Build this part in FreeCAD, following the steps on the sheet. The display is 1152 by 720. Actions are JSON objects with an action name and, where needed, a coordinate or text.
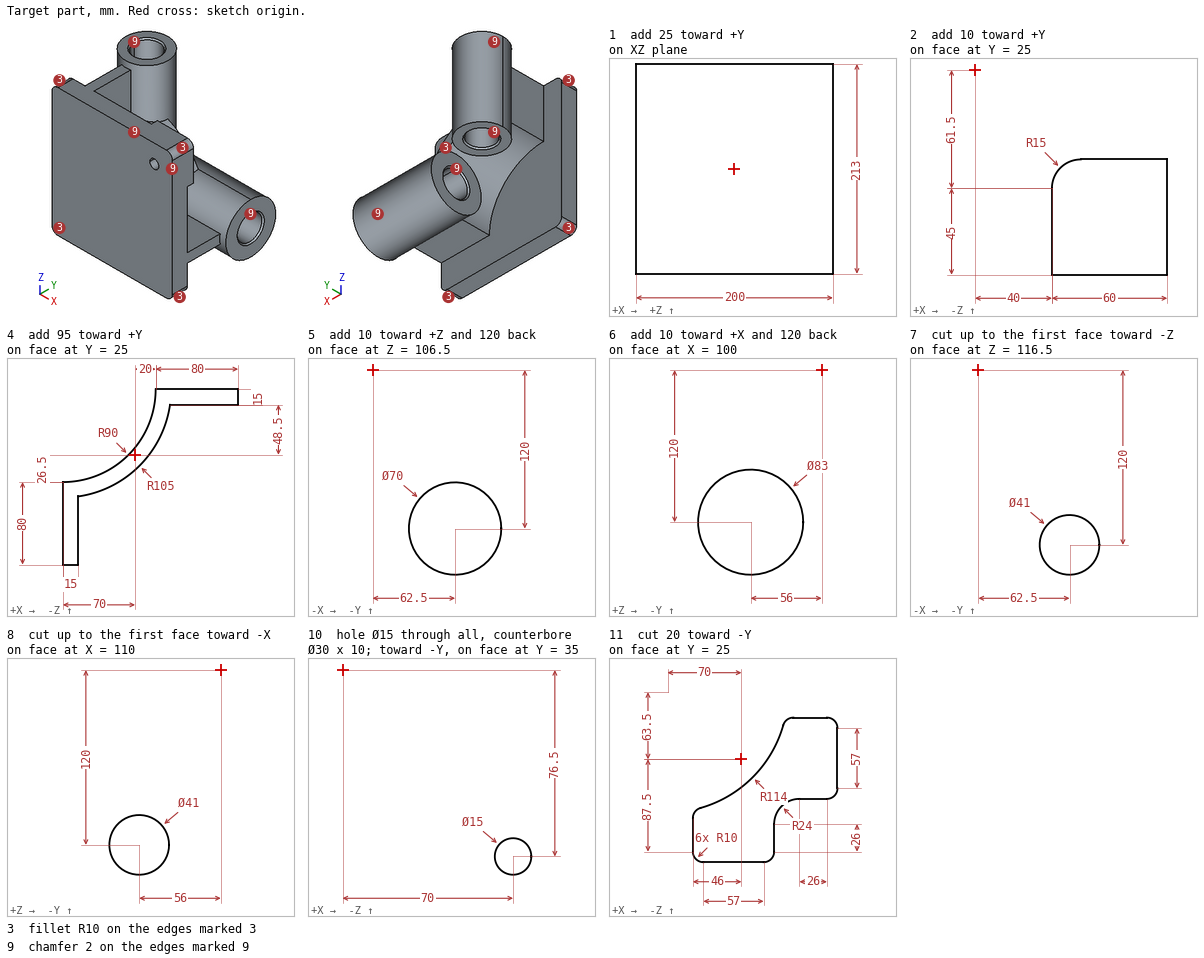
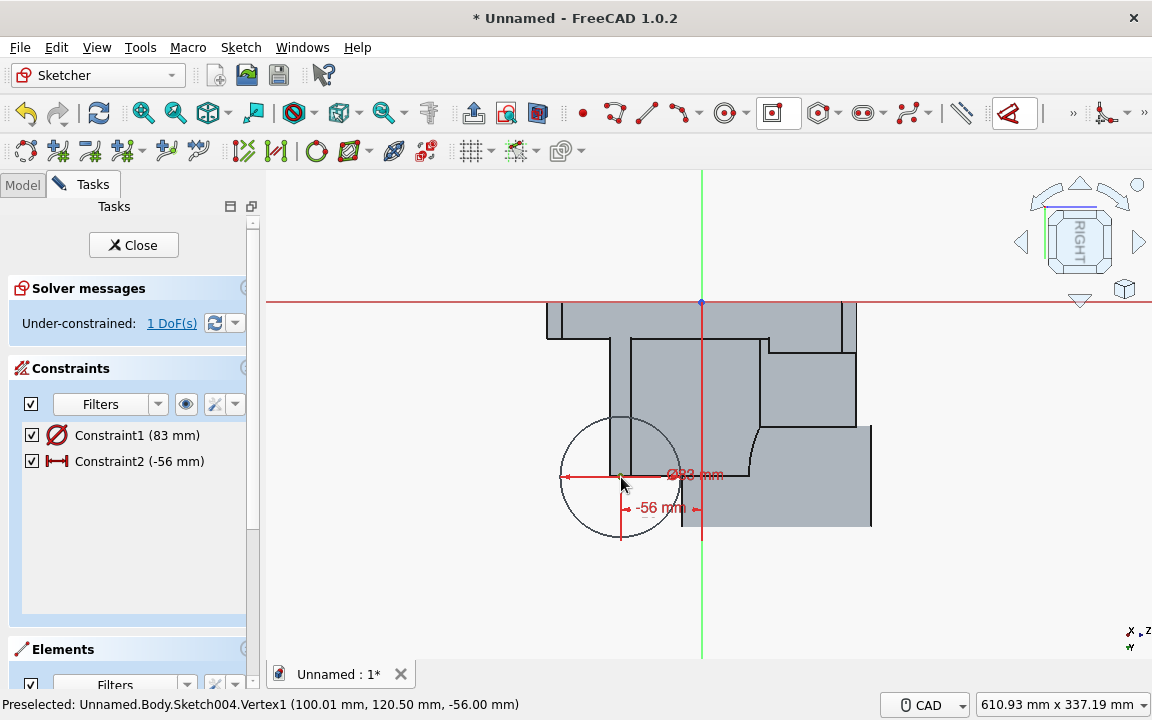
{"action": "key", "text": "i"}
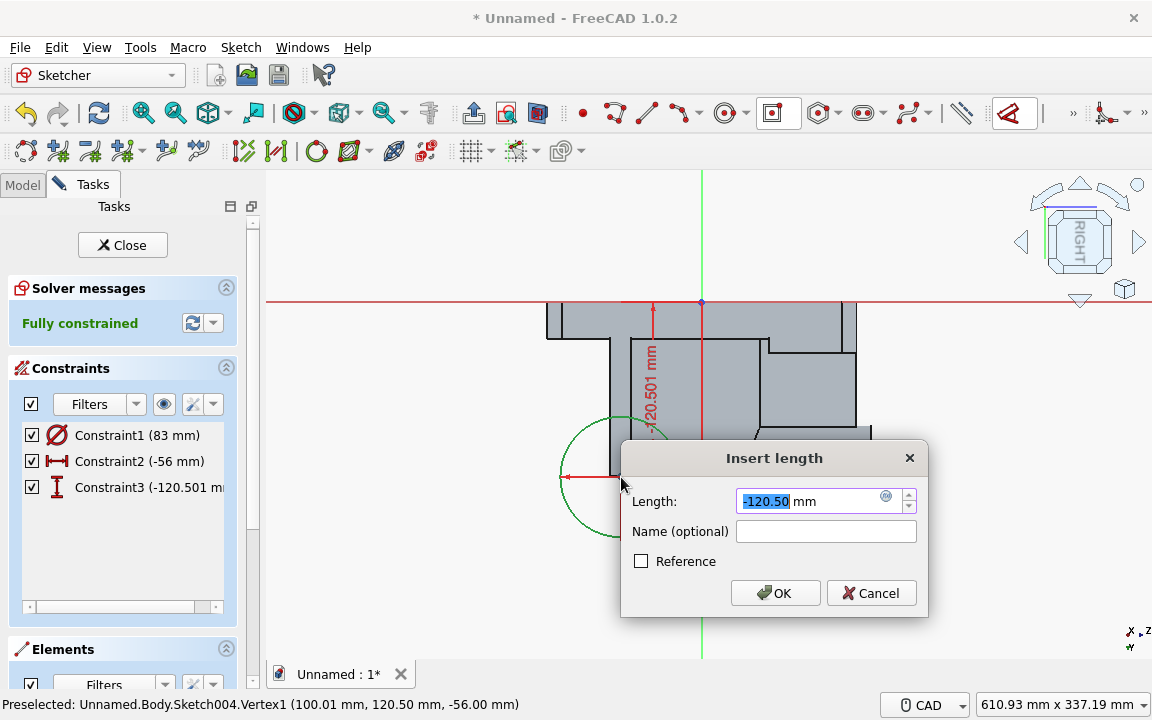
{"action": "type", "text": "-120"}
{"action": "key", "text": "Return"}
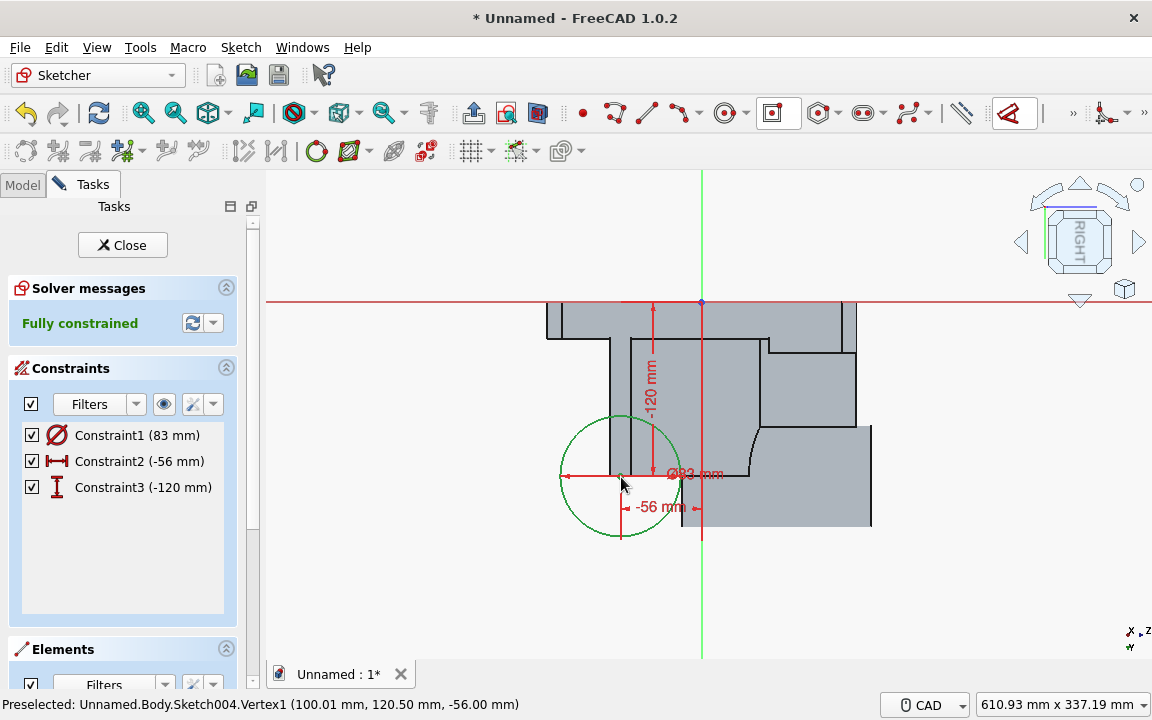
{"action": "left_click", "coordinate": [123, 245]}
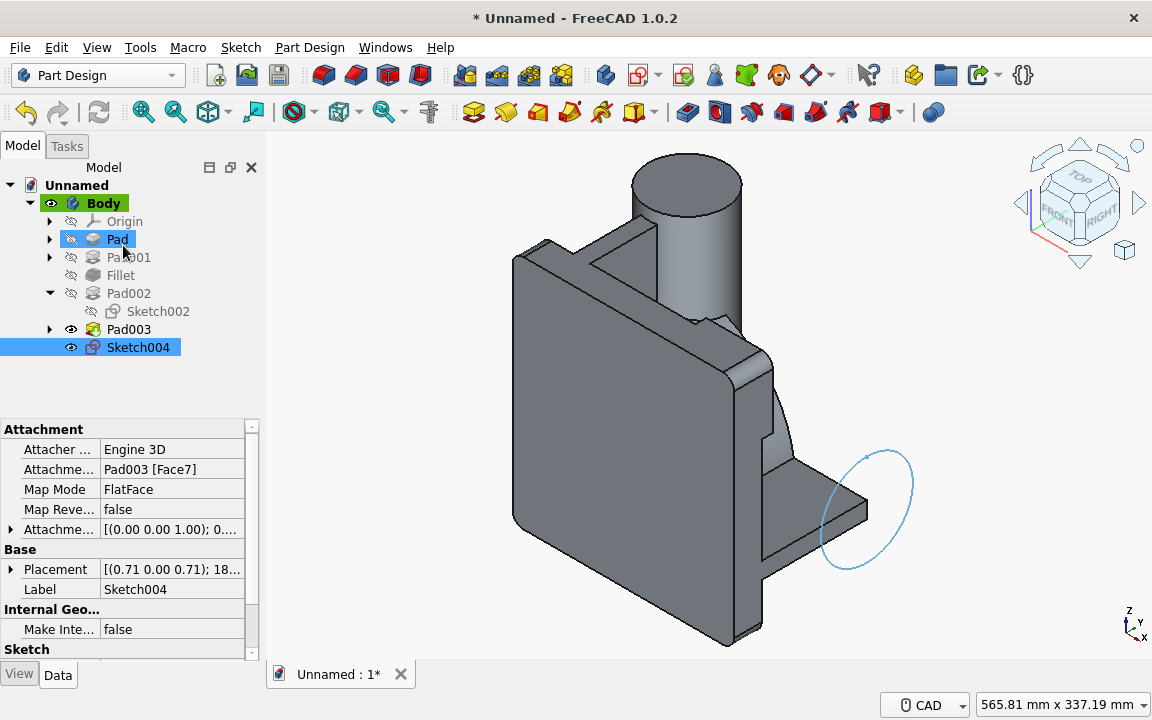
{"action": "left_click", "coordinate": [474, 112]}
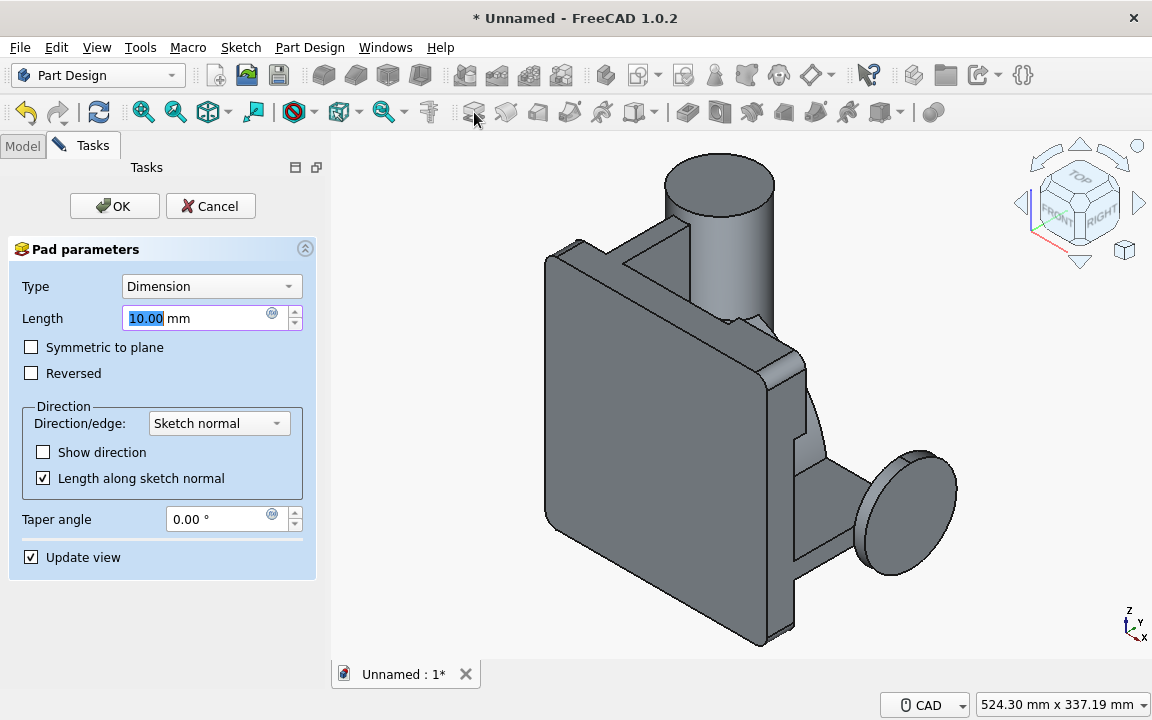
{"action": "left_click", "coordinate": [212, 286]}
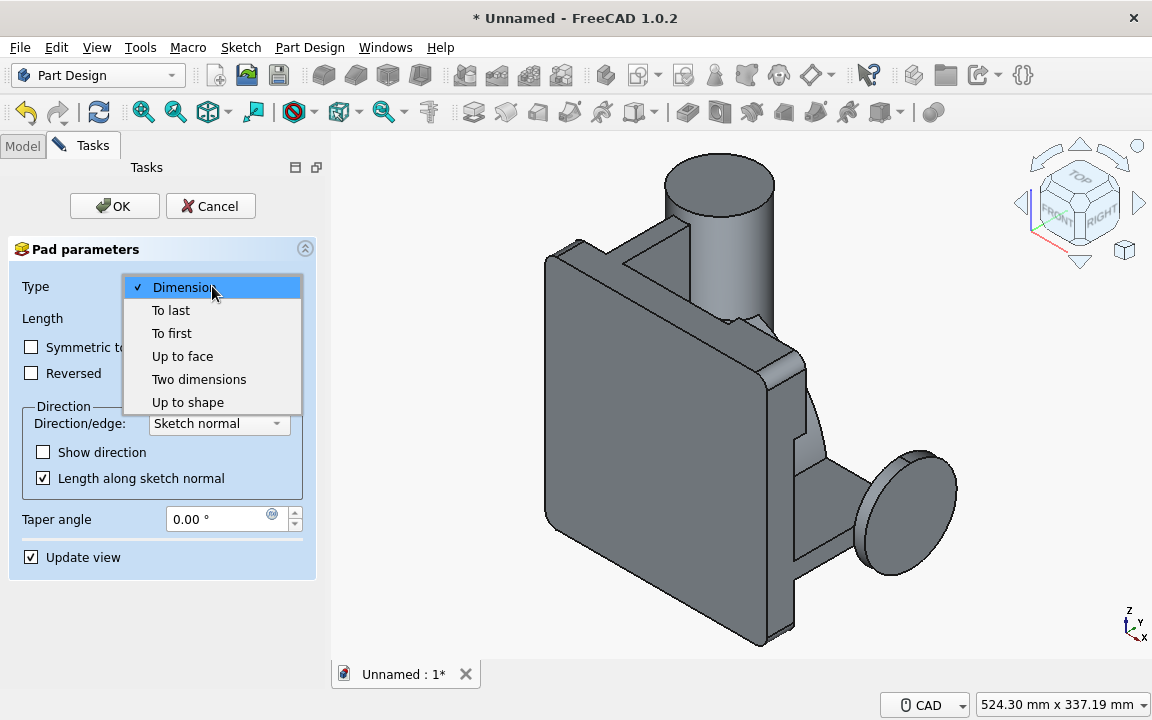
{"action": "left_click", "coordinate": [212, 380]}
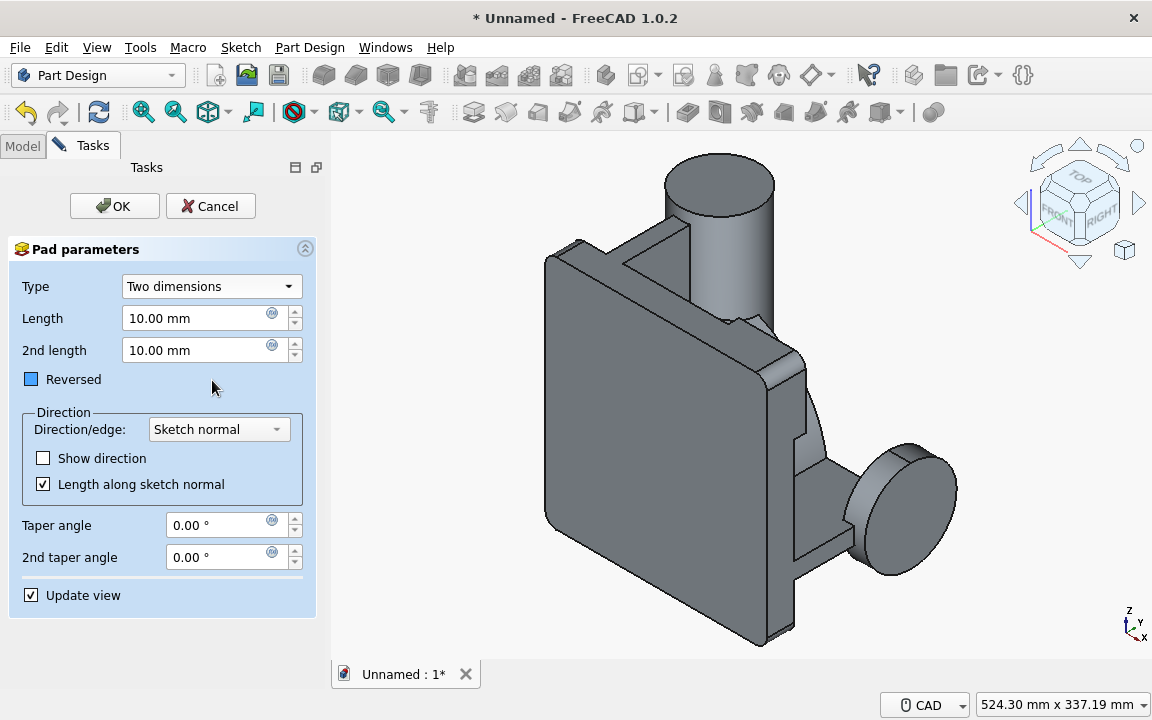
{"action": "triple_click", "coordinate": [204, 318]}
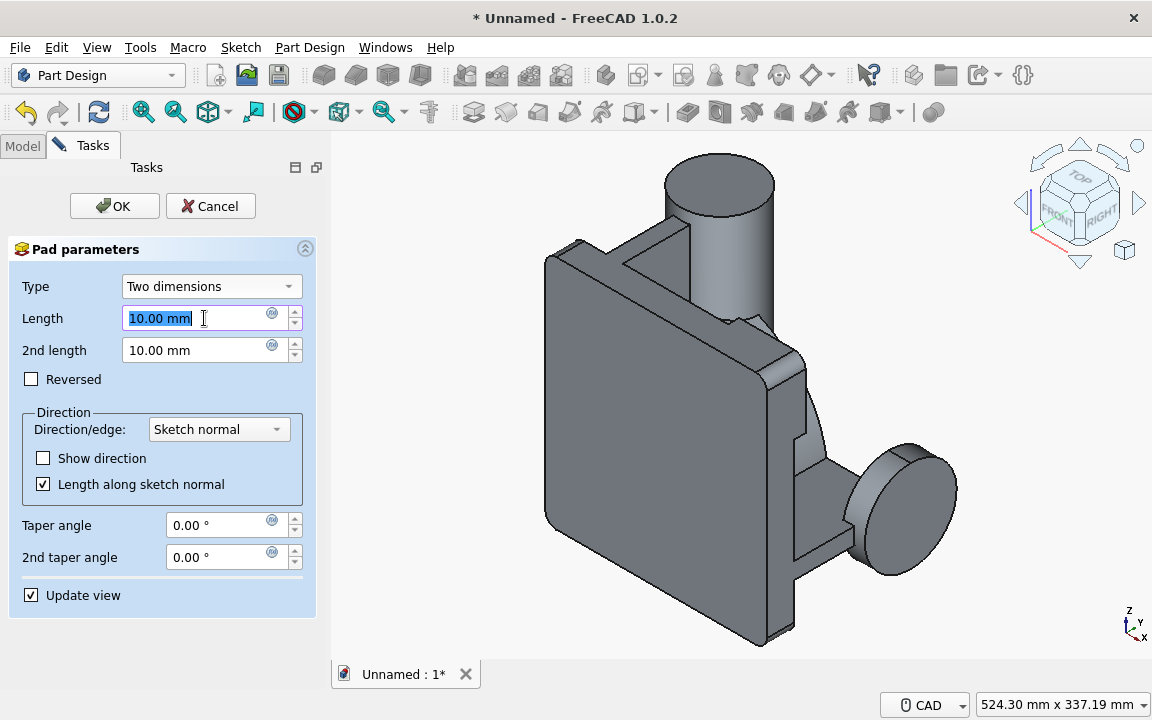
{"action": "type", "text": "10"}
{"action": "key", "text": "Tab"}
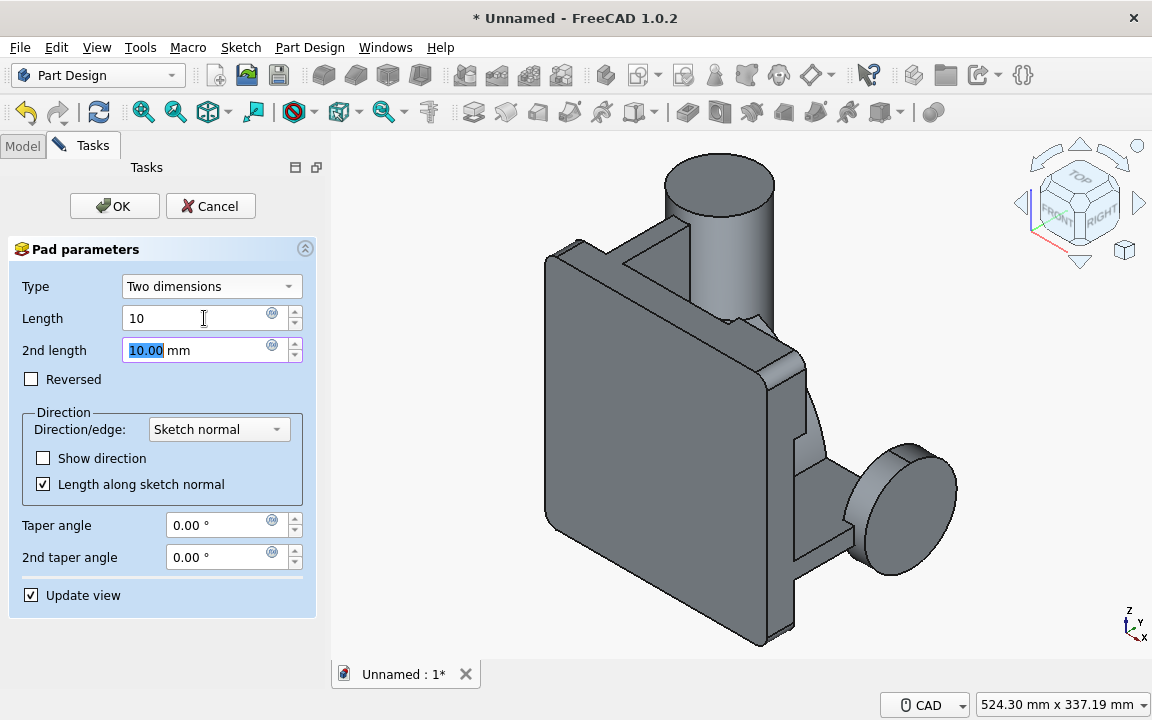
{"action": "type", "text": "120"}
{"action": "key", "text": "Tab"}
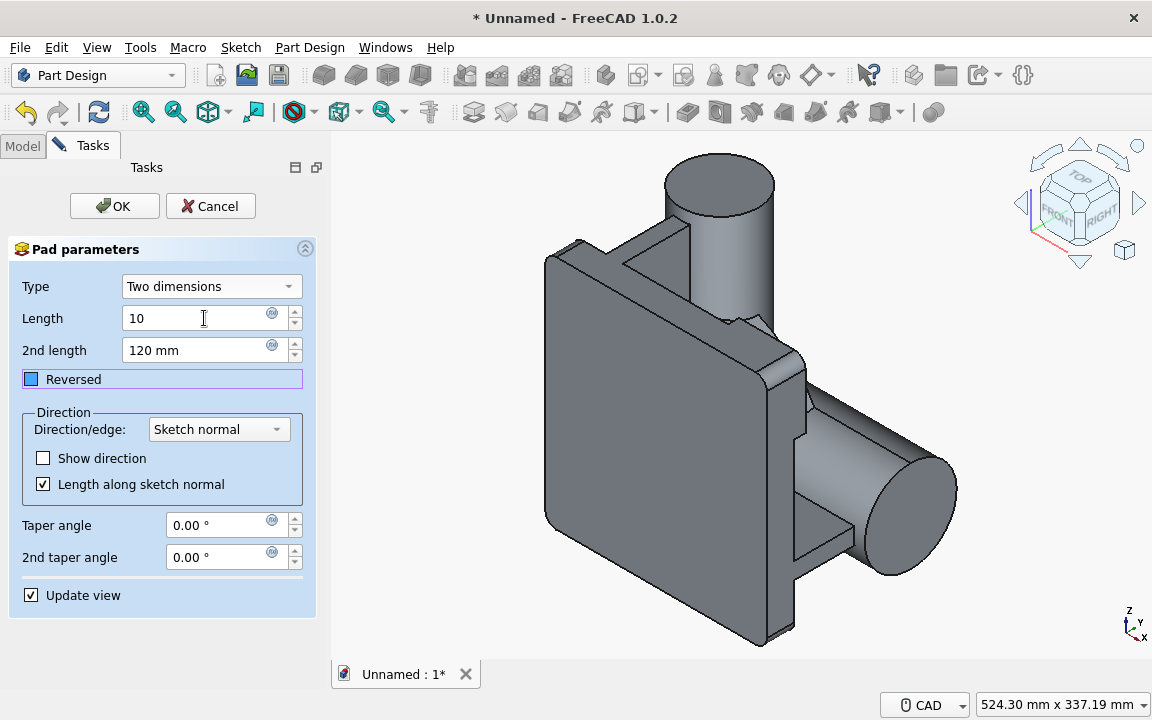
{"action": "left_click", "coordinate": [115, 206]}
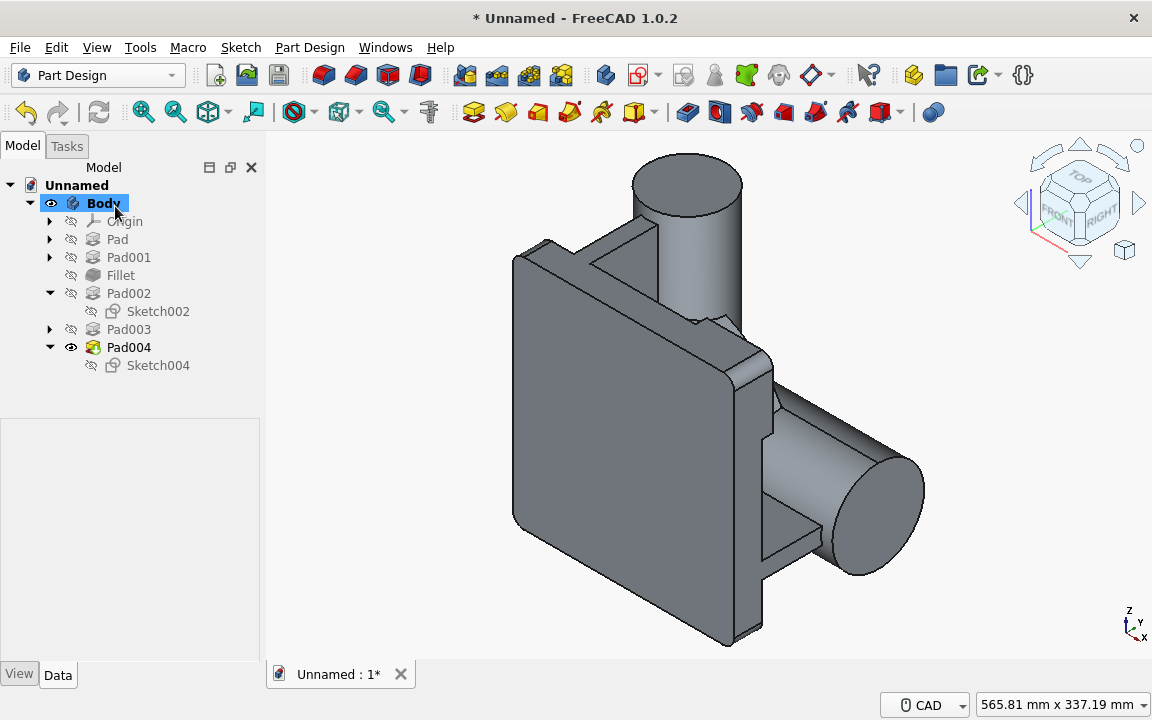
{"action": "left_click", "coordinate": [687, 184]}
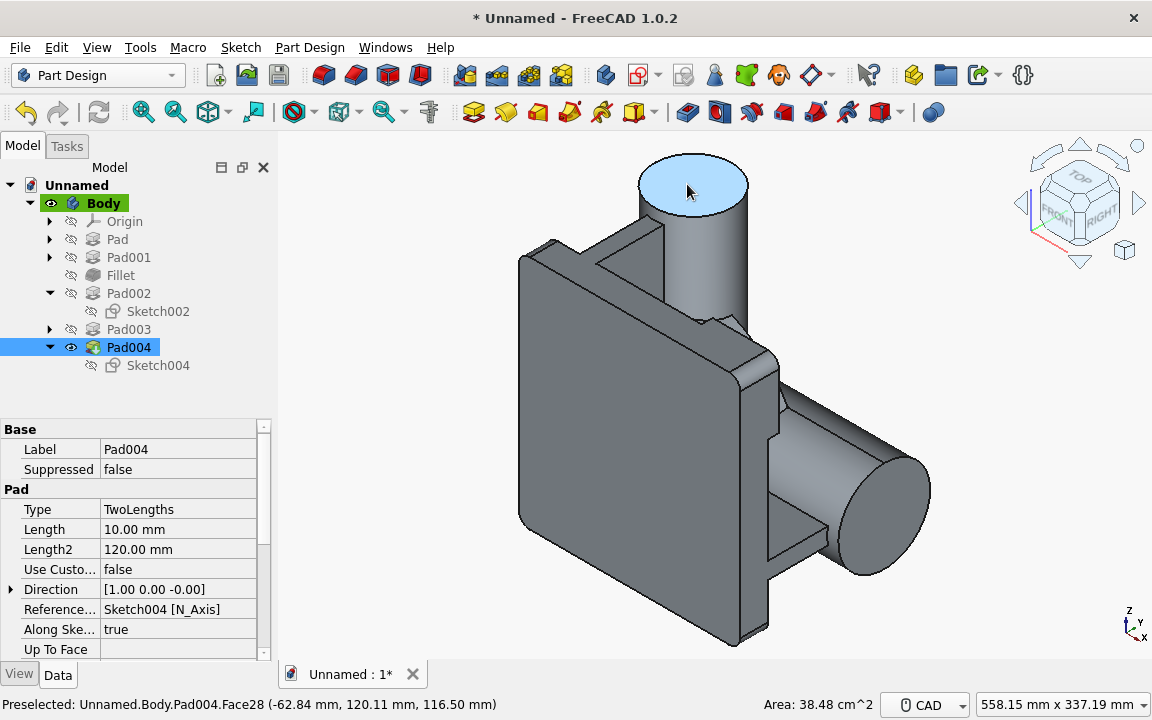
{"action": "left_click", "coordinate": [638, 76]}